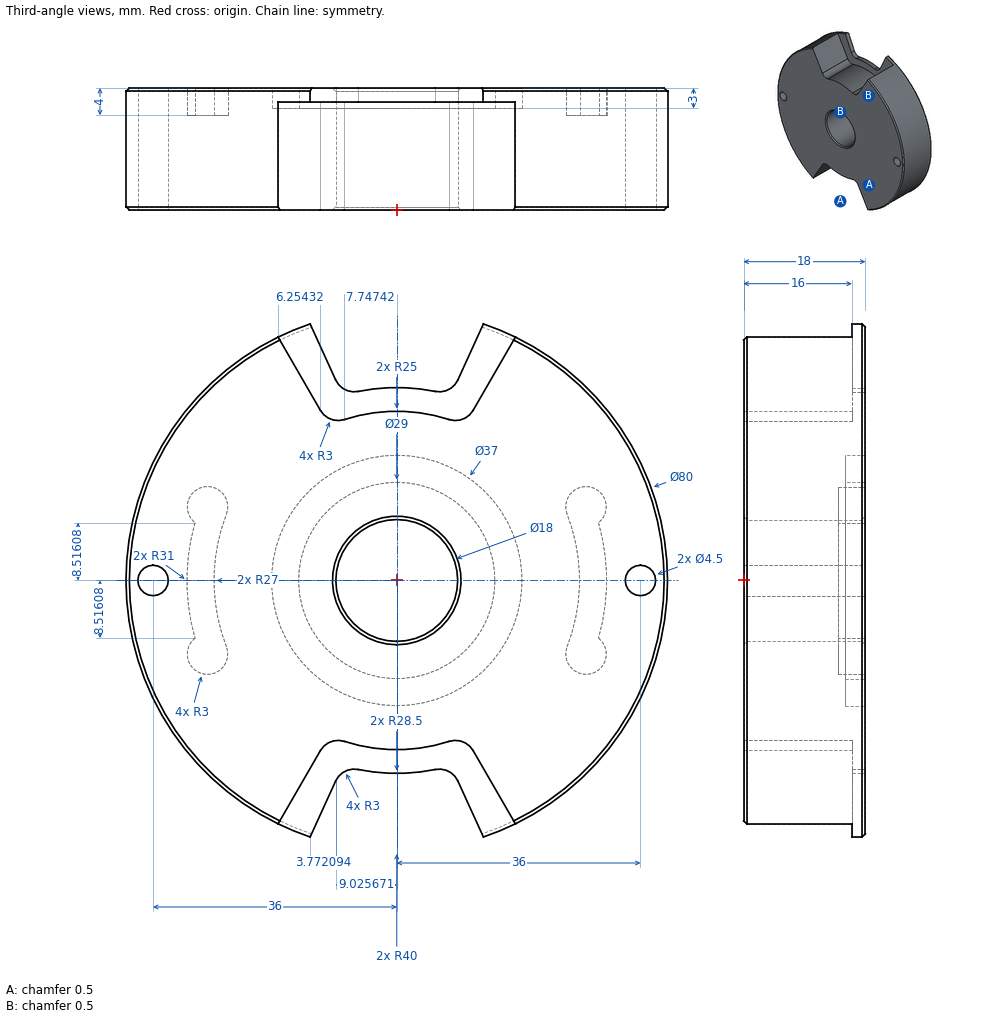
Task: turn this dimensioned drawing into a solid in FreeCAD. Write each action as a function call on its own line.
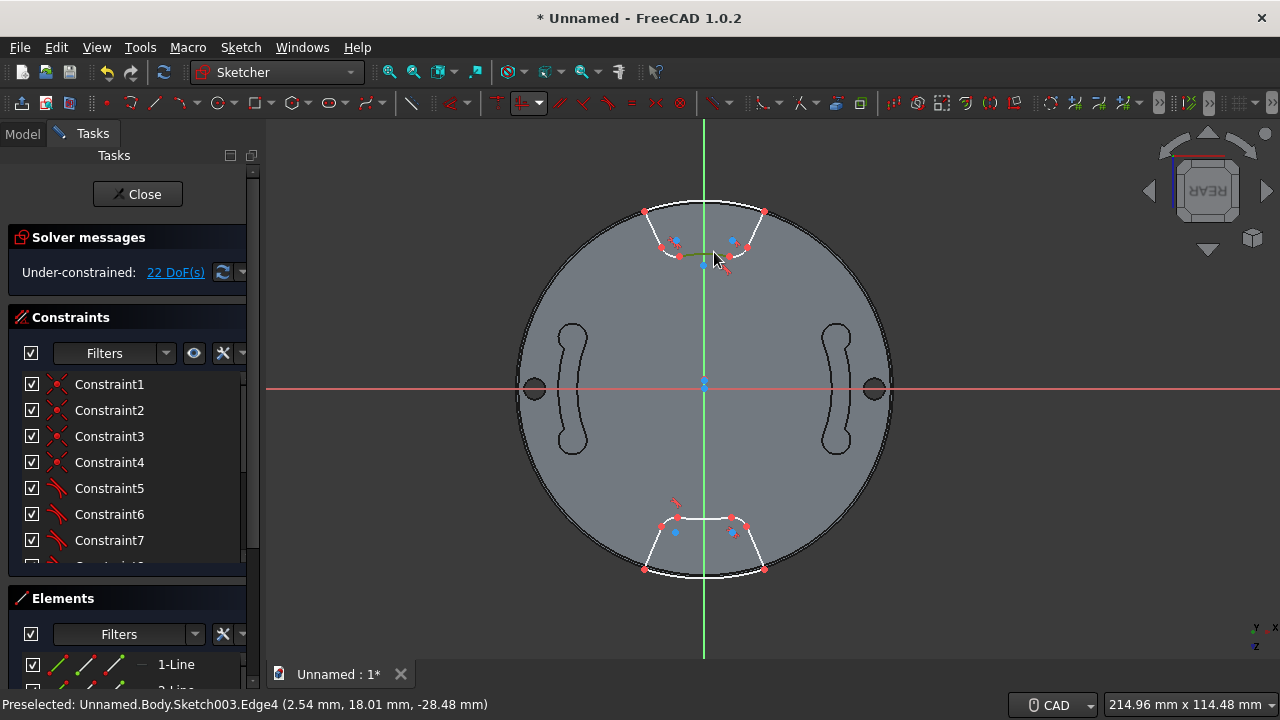
scroll(693, 519, up, 2)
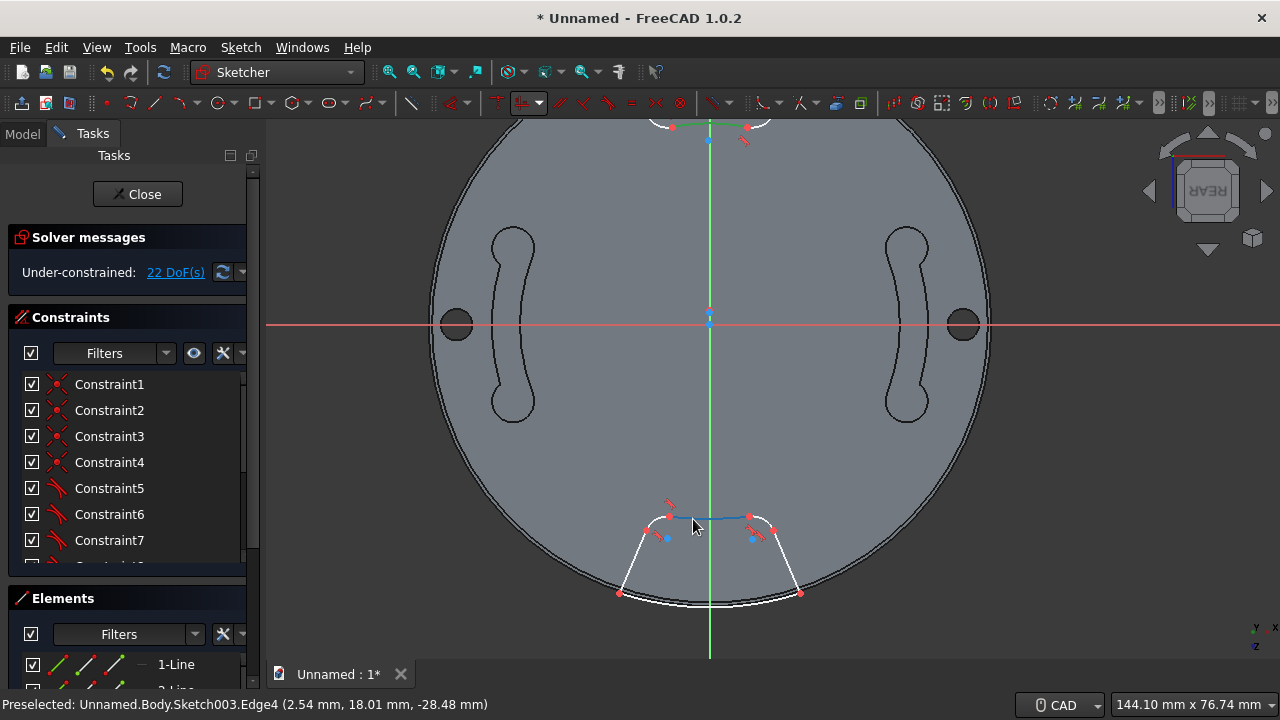
click(693, 518)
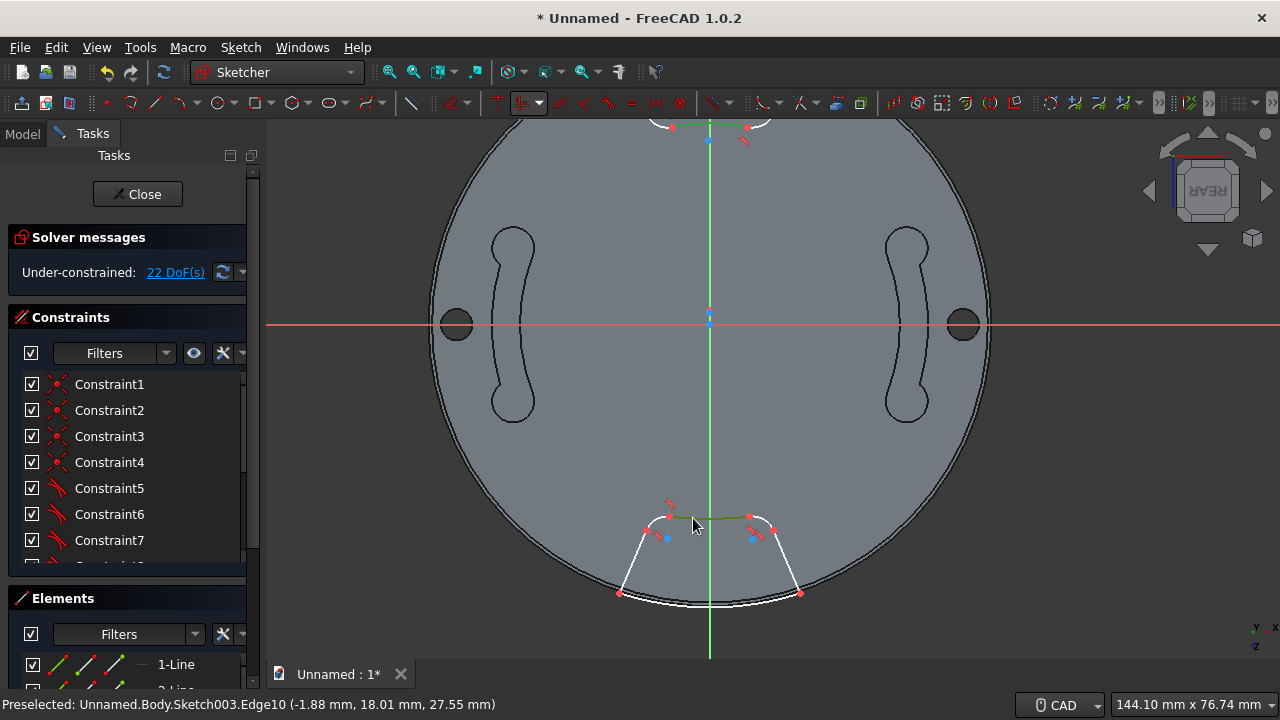
click(498, 104)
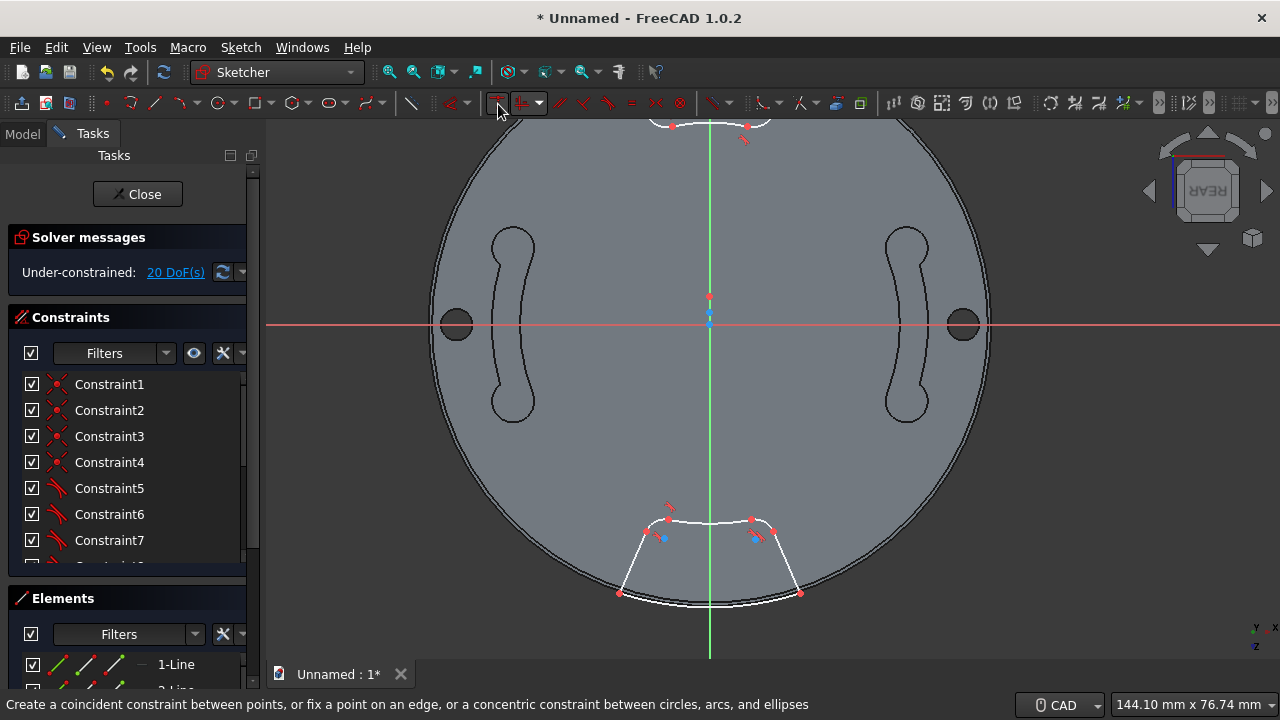
scroll(693, 520, down, 2)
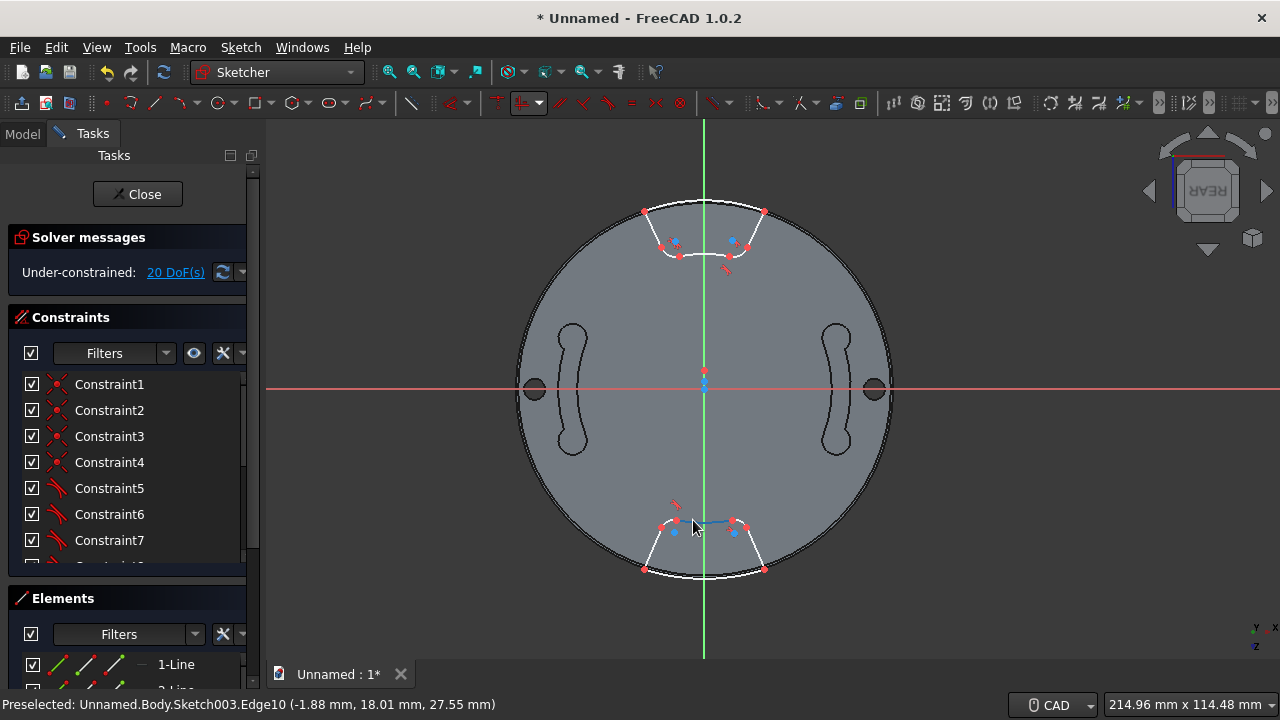
scroll(714, 254, up, 2)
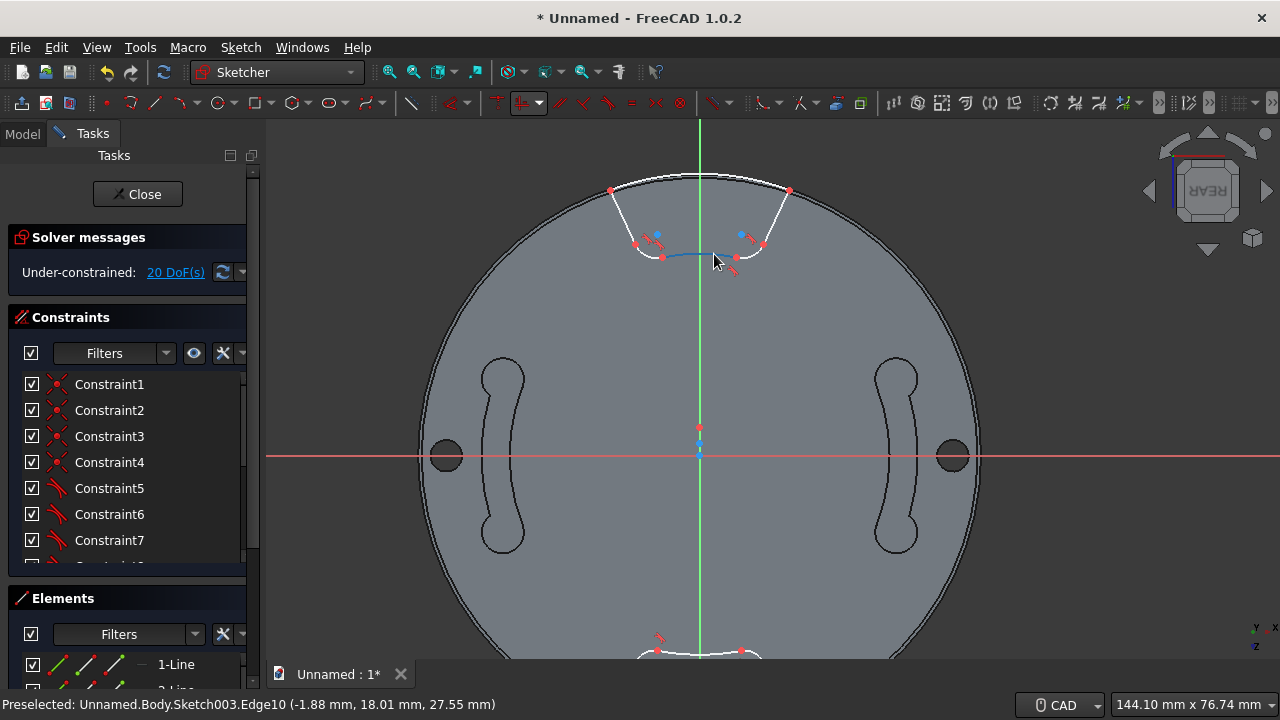
click(715, 254)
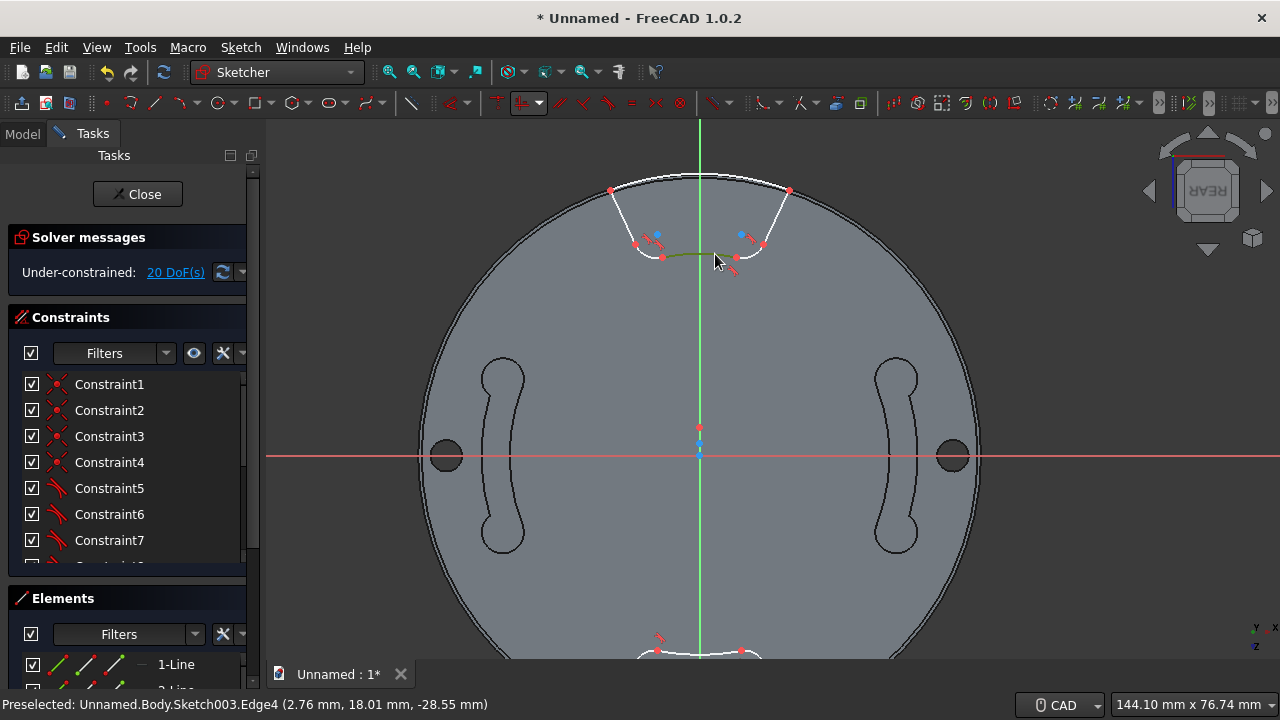
scroll(714, 253, down, 2)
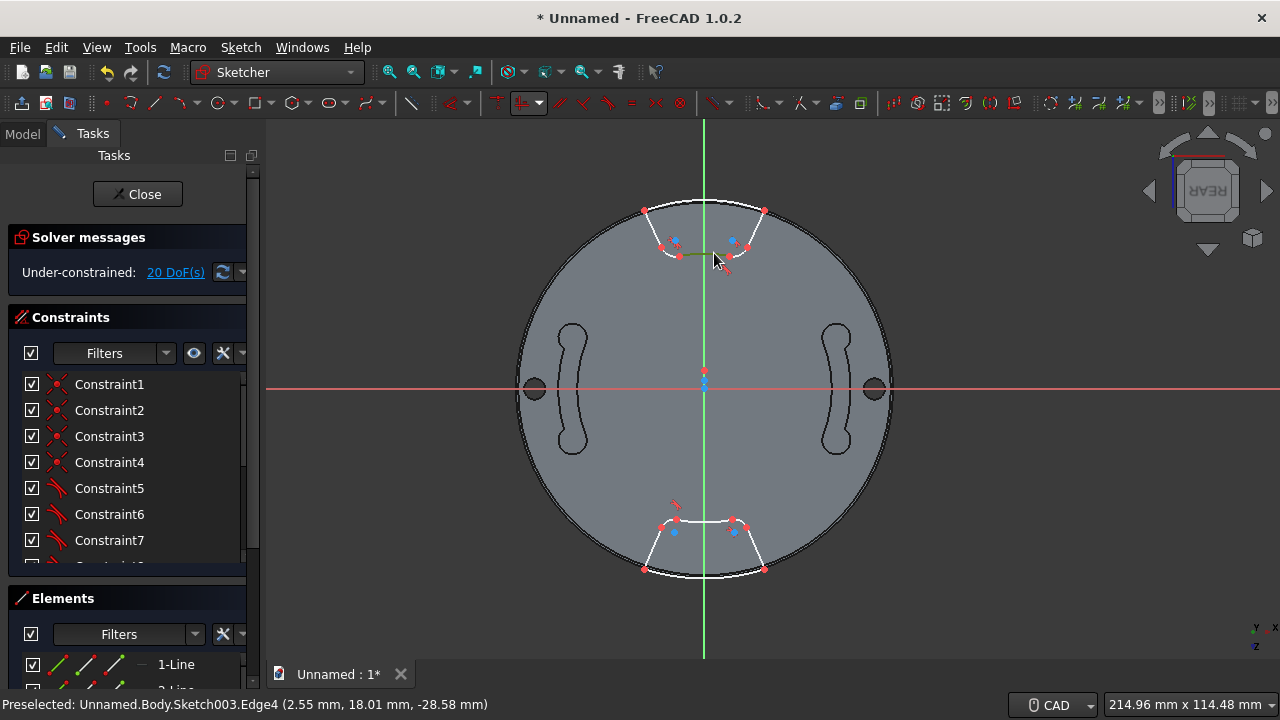
click(680, 577)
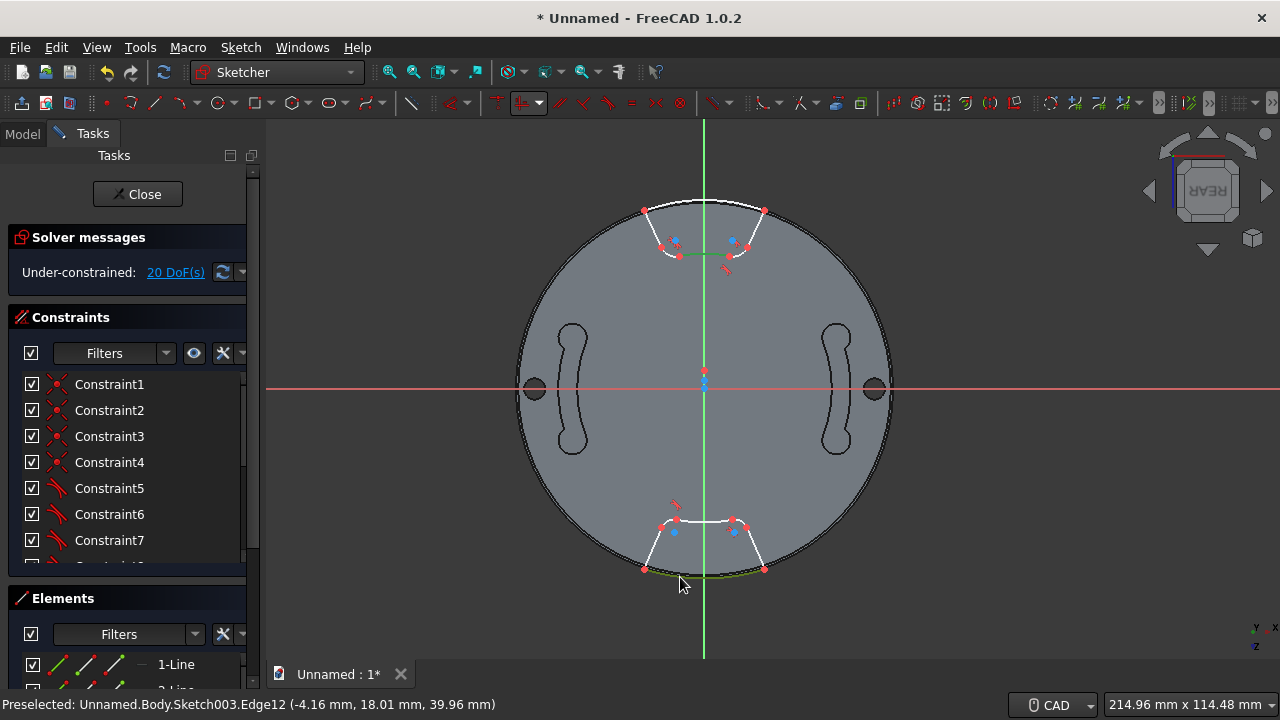
click(498, 104)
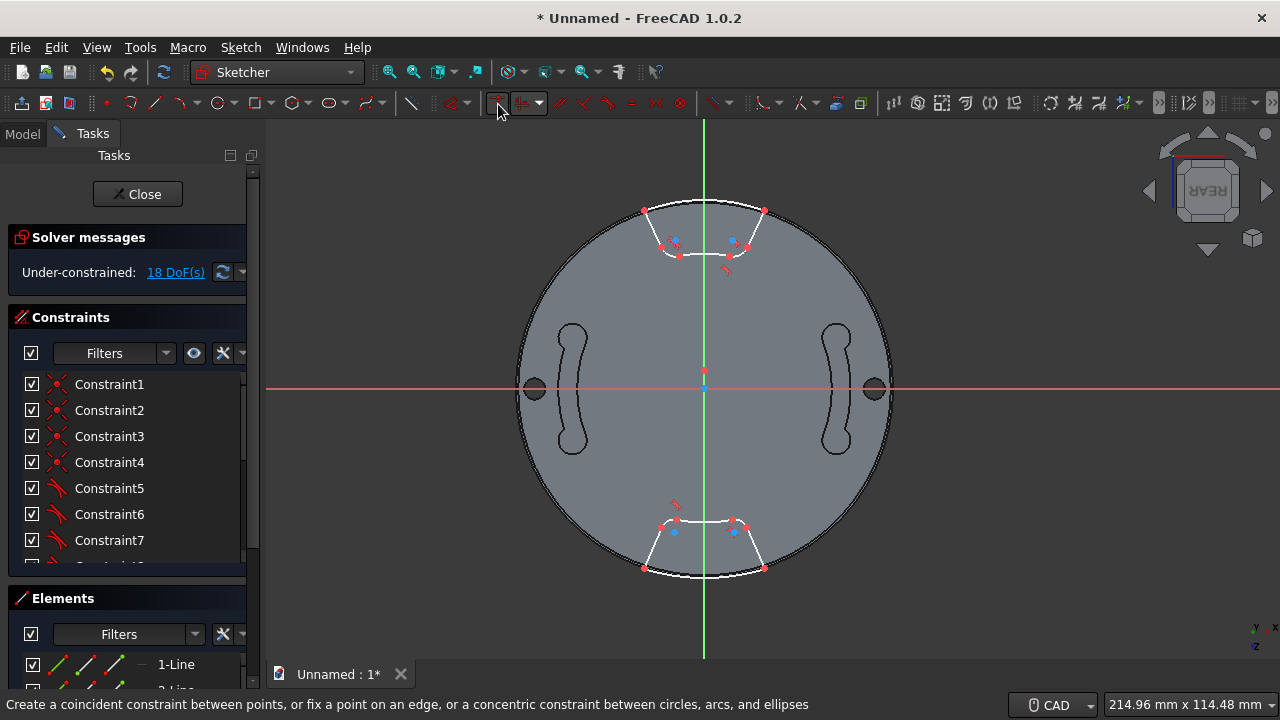
scroll(704, 380, up, 6)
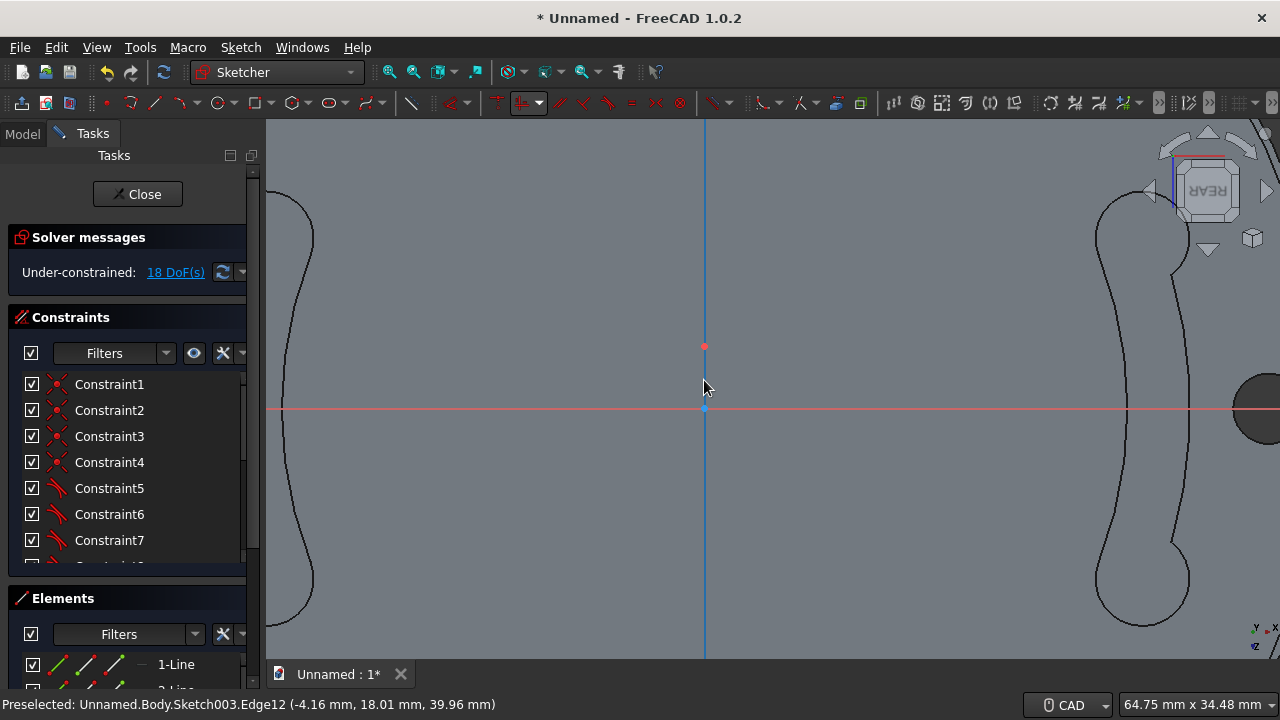
drag(695, 336, 715, 419)